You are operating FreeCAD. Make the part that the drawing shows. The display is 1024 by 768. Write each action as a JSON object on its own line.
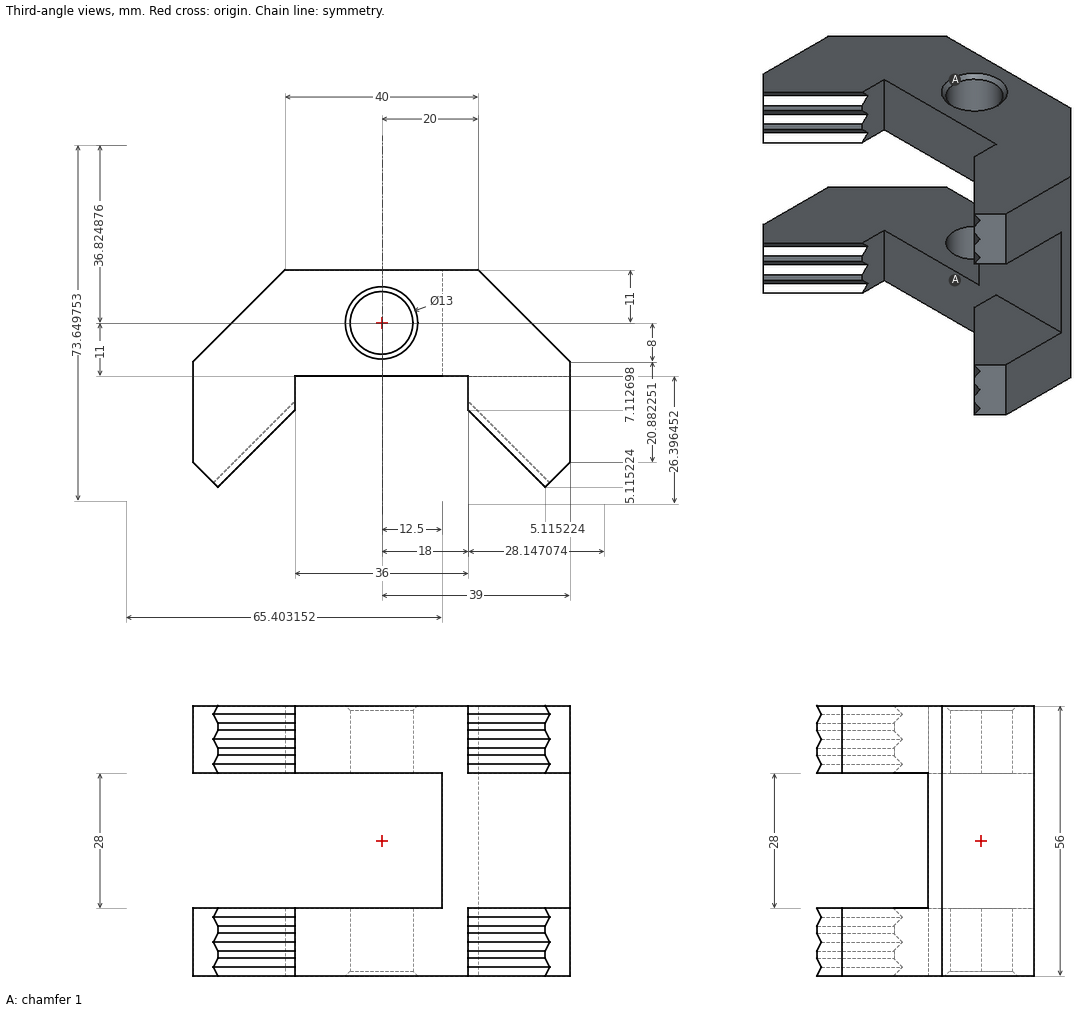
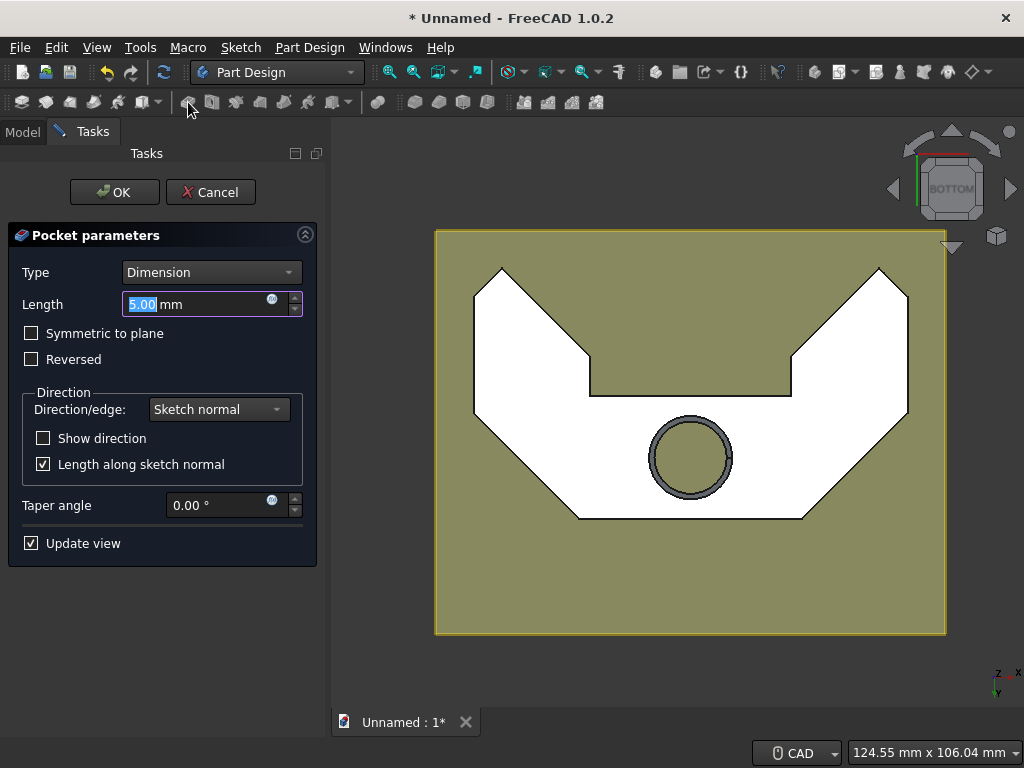
{"action": "type", "text": "28"}
{"action": "key", "text": "Tab"}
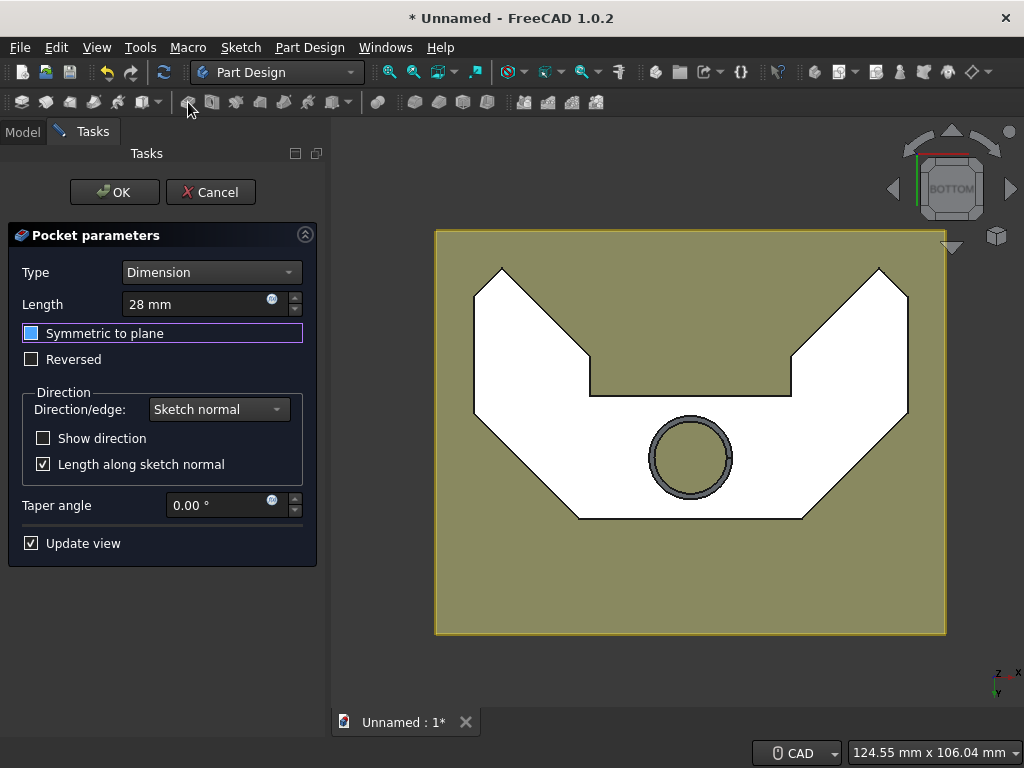
{"action": "left_click", "coordinate": [115, 192]}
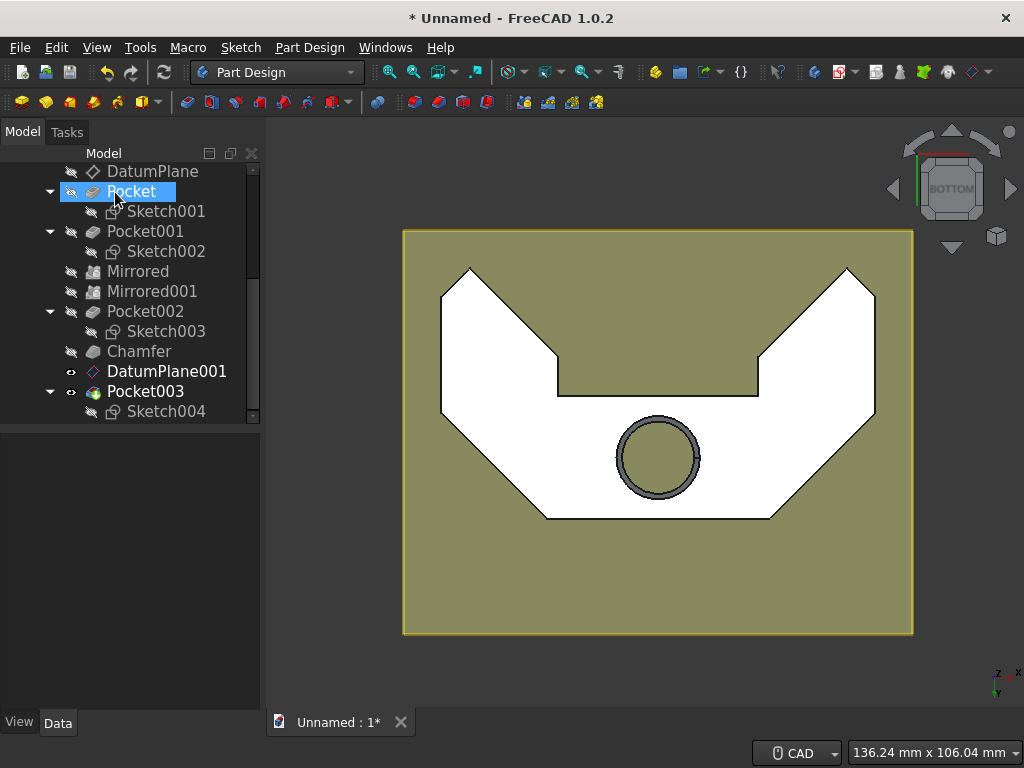
{"action": "left_click", "coordinate": [116, 372]}
{"action": "key", "text": "space"}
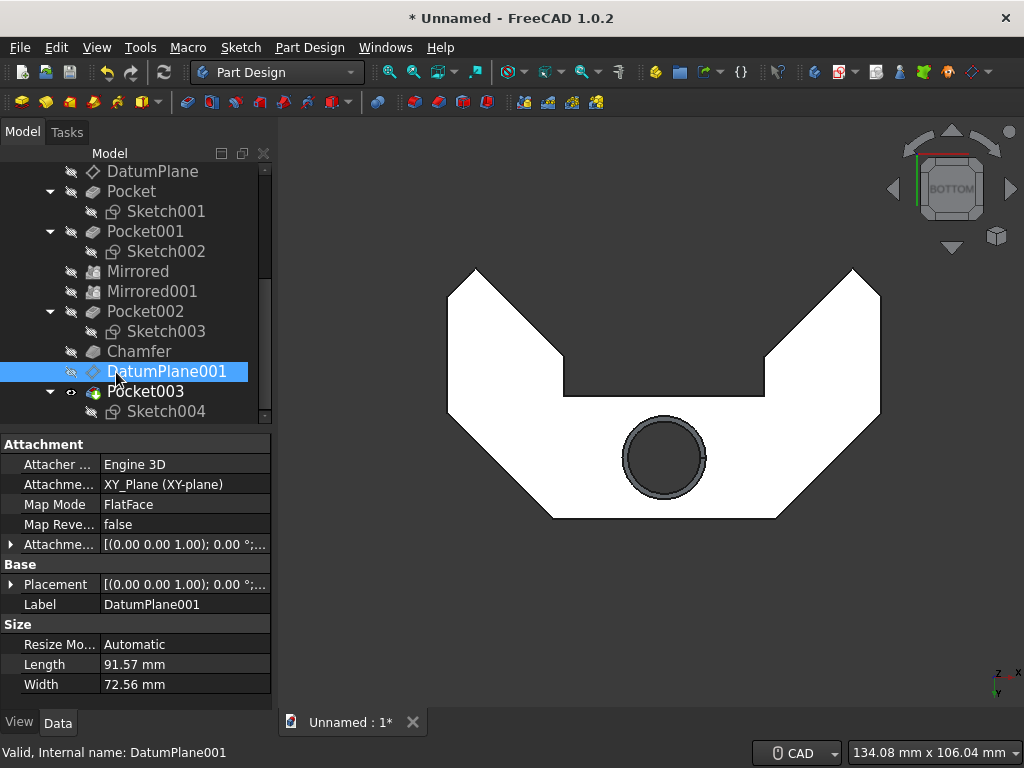
{"action": "key", "text": "0"}